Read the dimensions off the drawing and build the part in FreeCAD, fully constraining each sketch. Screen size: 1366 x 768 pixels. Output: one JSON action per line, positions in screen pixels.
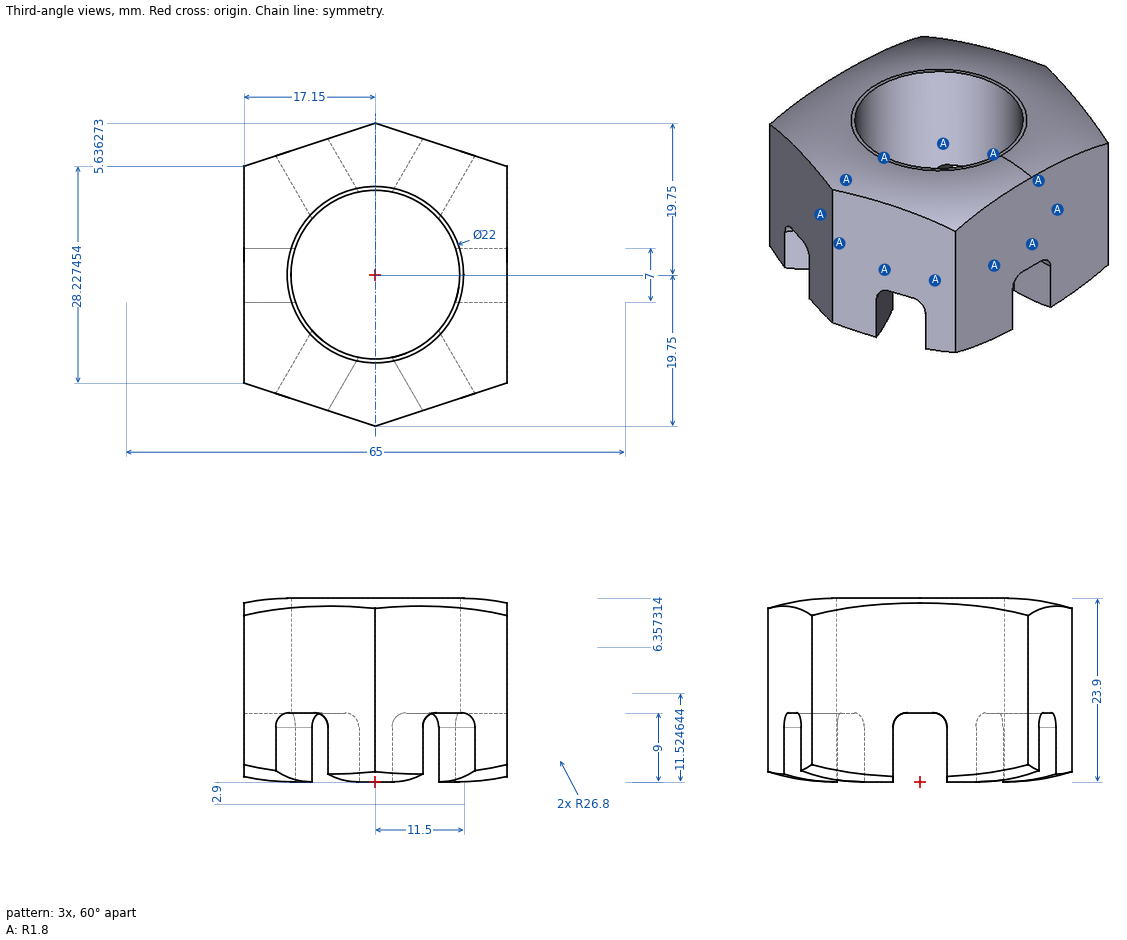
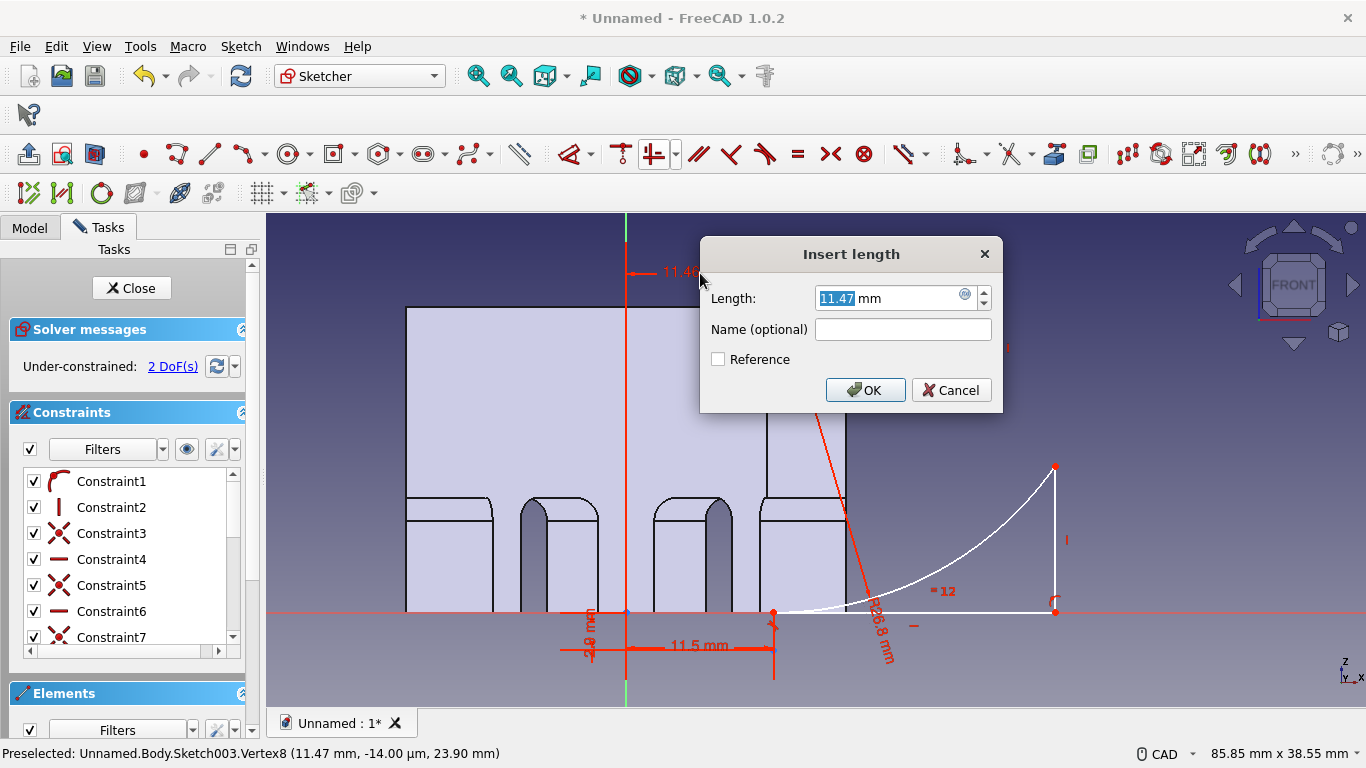
{"action": "type", "text": "11.5"}
{"action": "key", "text": "Return"}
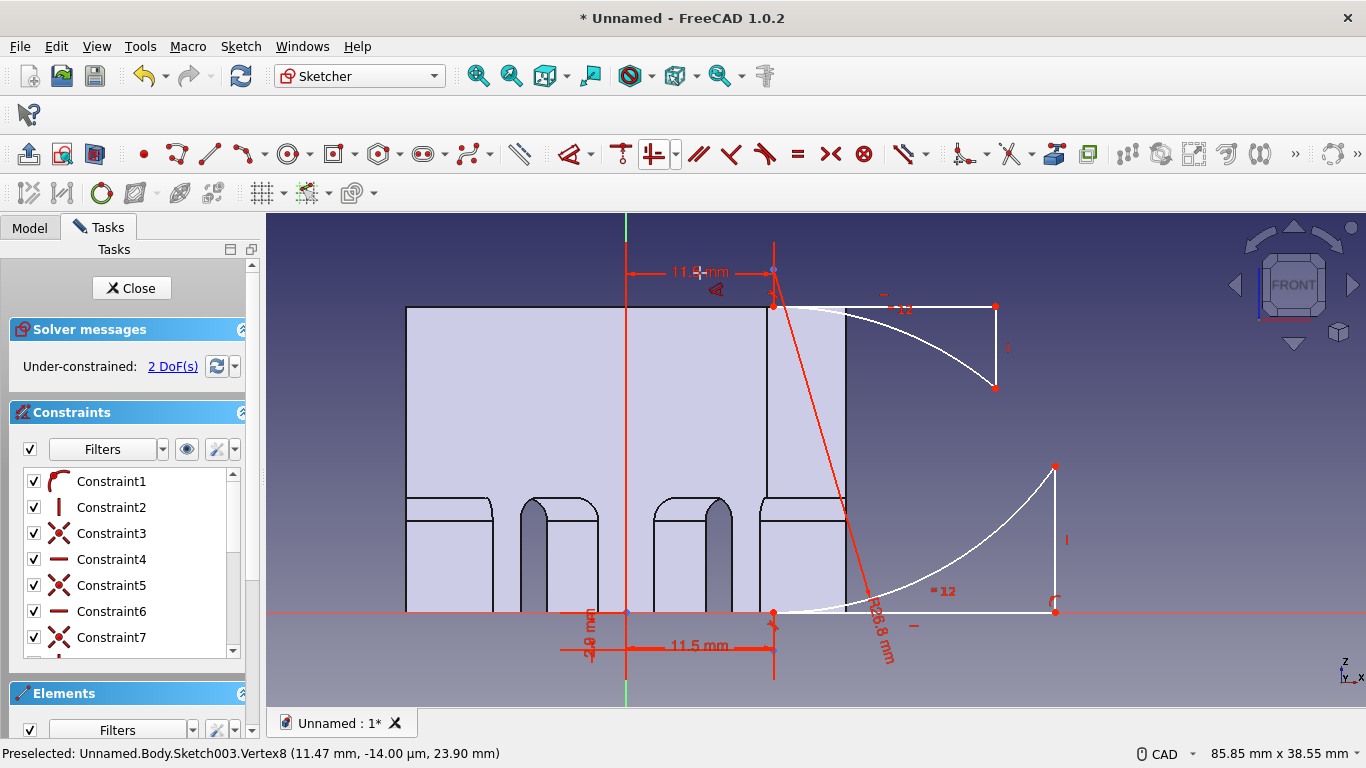
{"action": "left_click", "coordinate": [996, 331]}
{"action": "left_click", "coordinate": [1030, 347]}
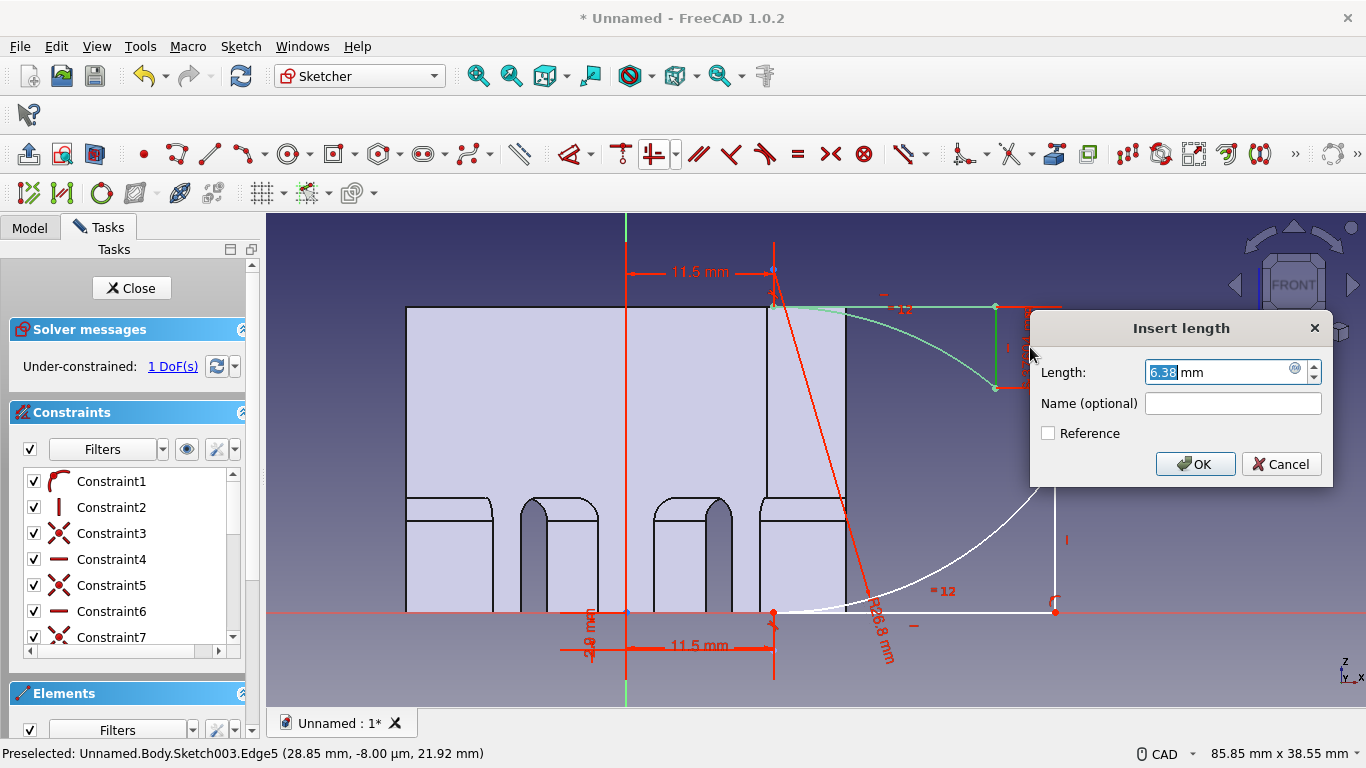
{"action": "type", "text": "6.357314"}
{"action": "key", "text": "Return"}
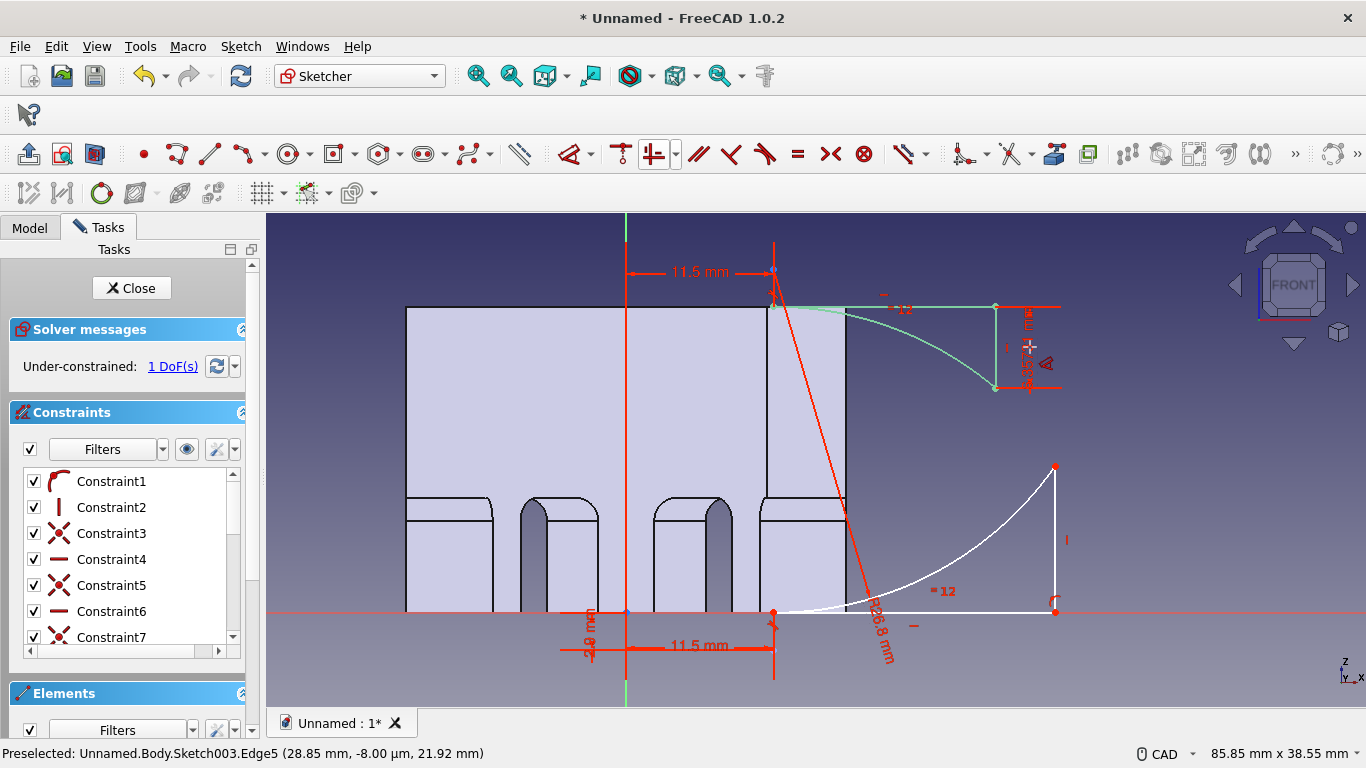
{"action": "left_click", "coordinate": [1055, 510]}
{"action": "left_click", "coordinate": [1089, 540]}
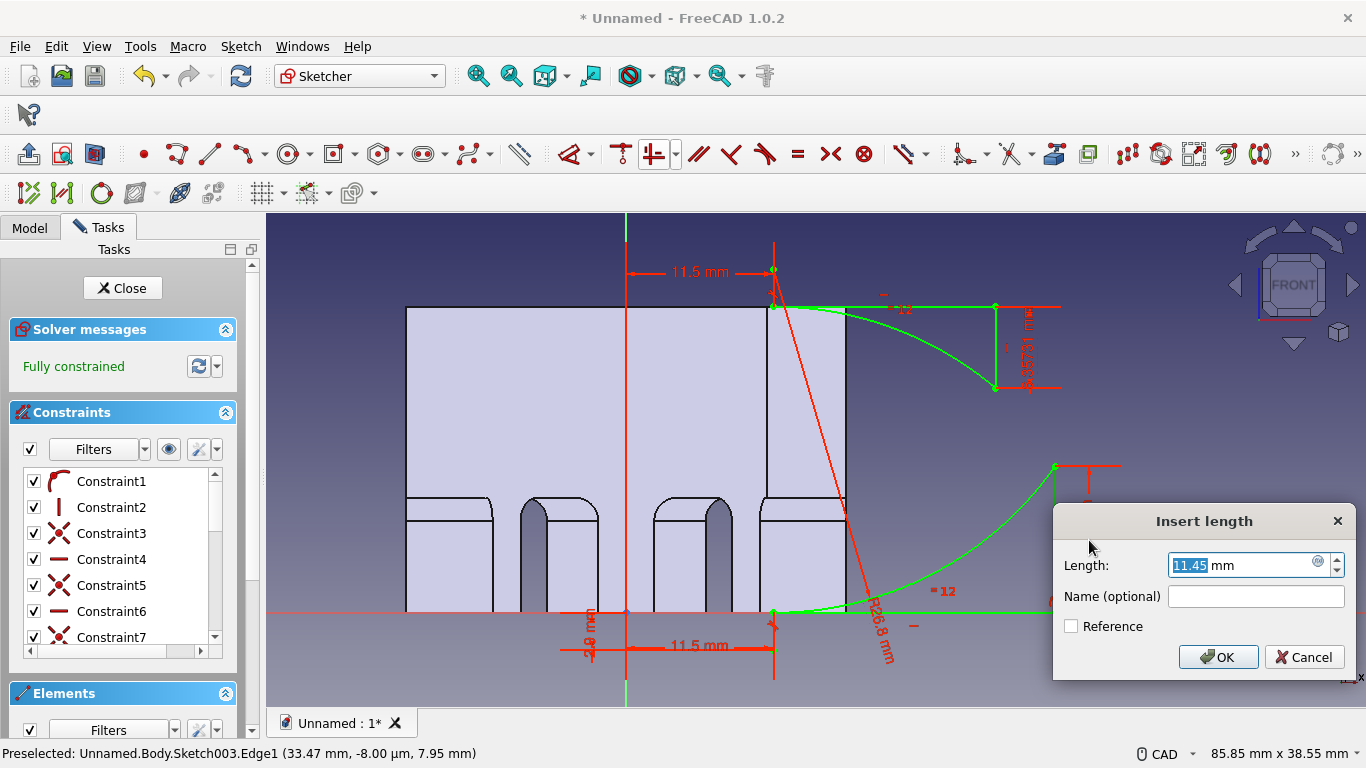
{"action": "type", "text": "11.524644"}
{"action": "key", "text": "Return"}
{"action": "key", "text": "Escape"}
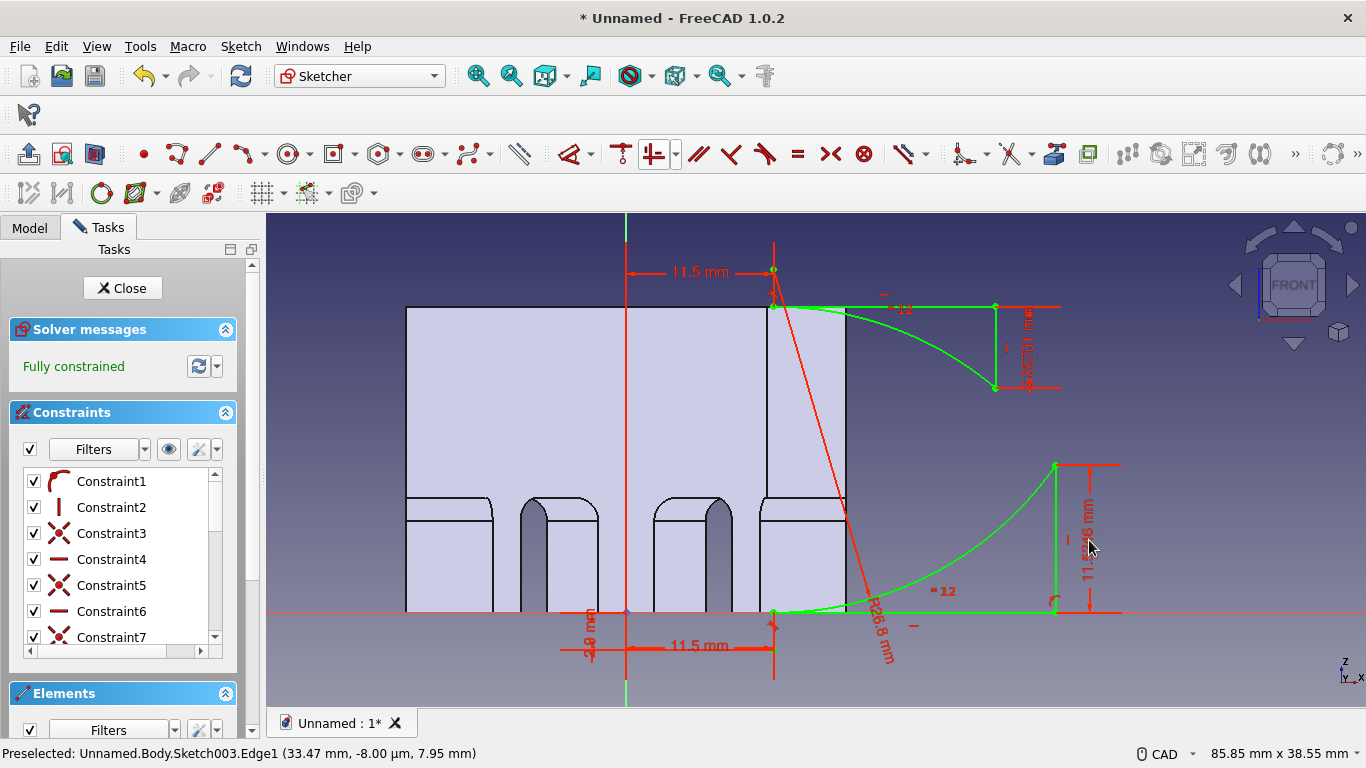
{"action": "left_click", "coordinate": [123, 288]}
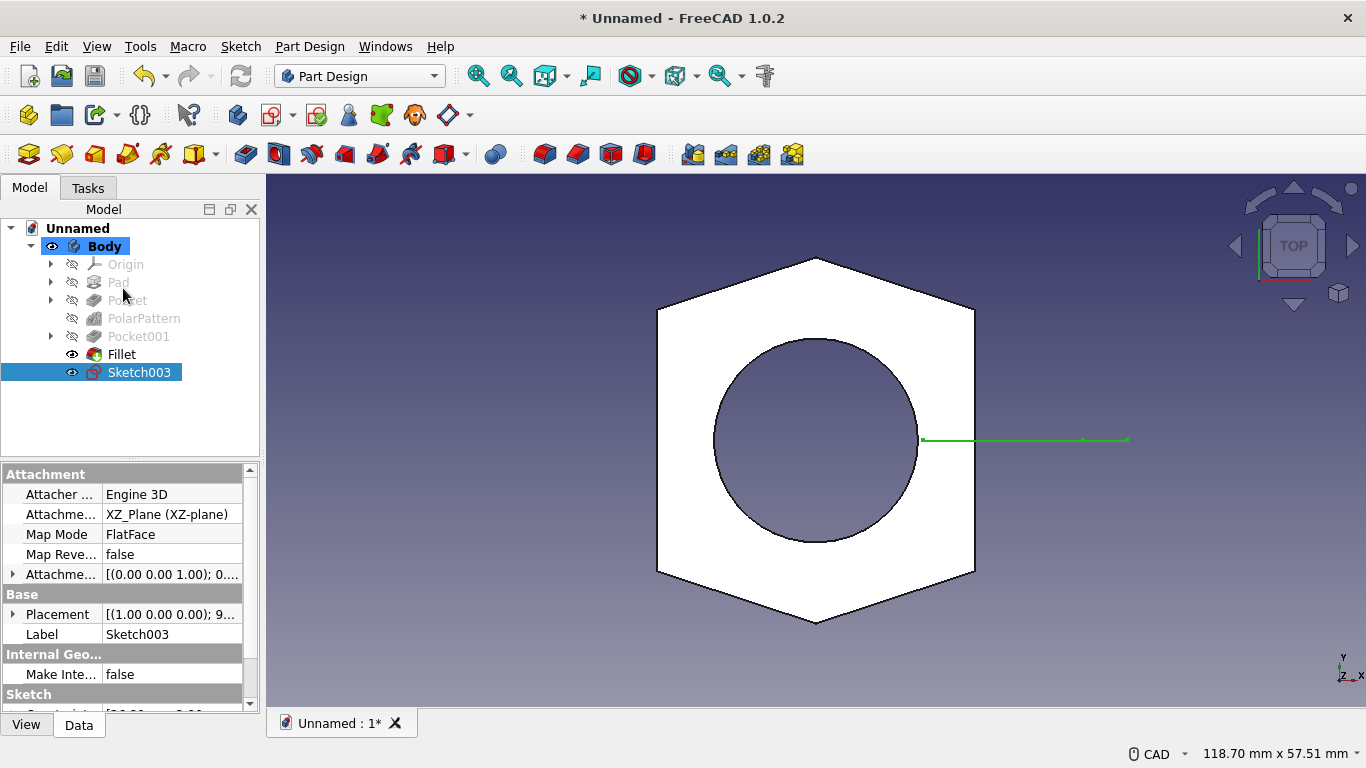
{"action": "left_click", "coordinate": [312, 154]}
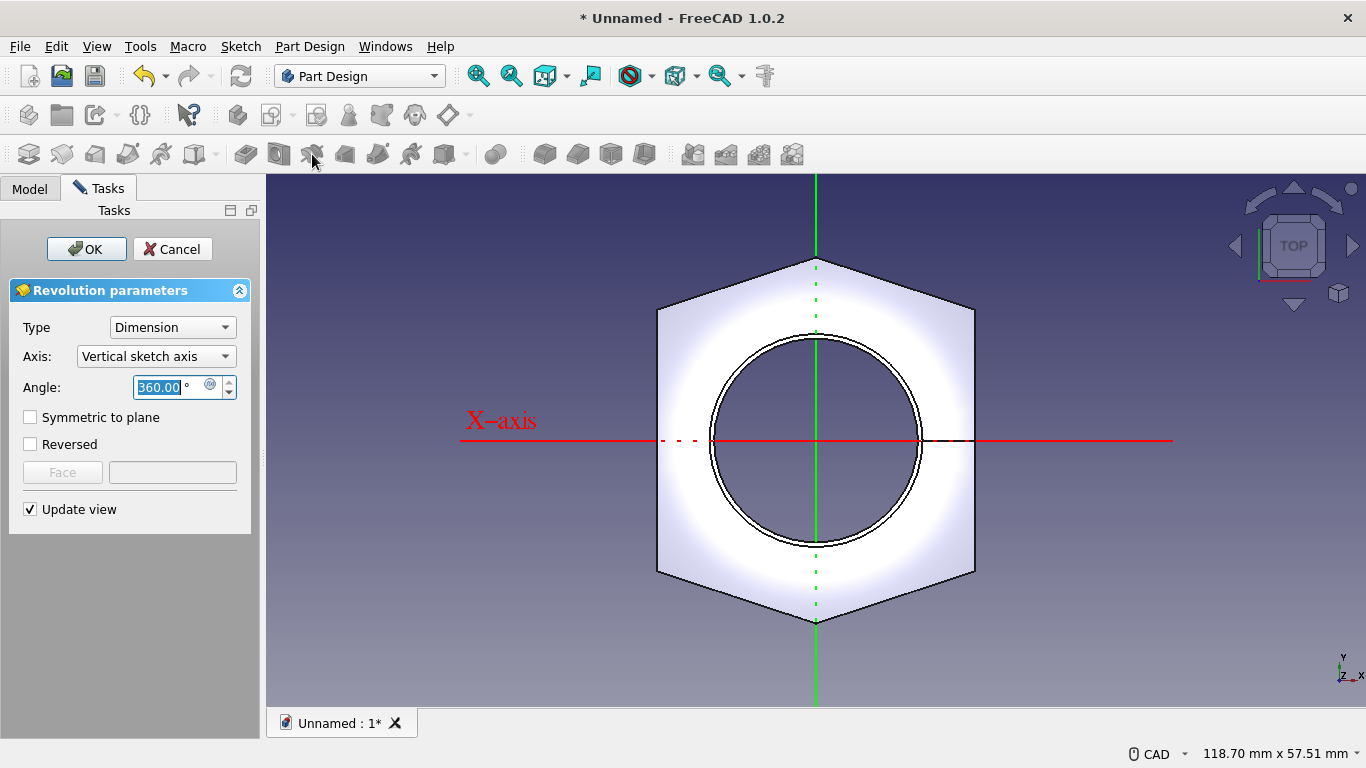
{"action": "left_click", "coordinate": [87, 249]}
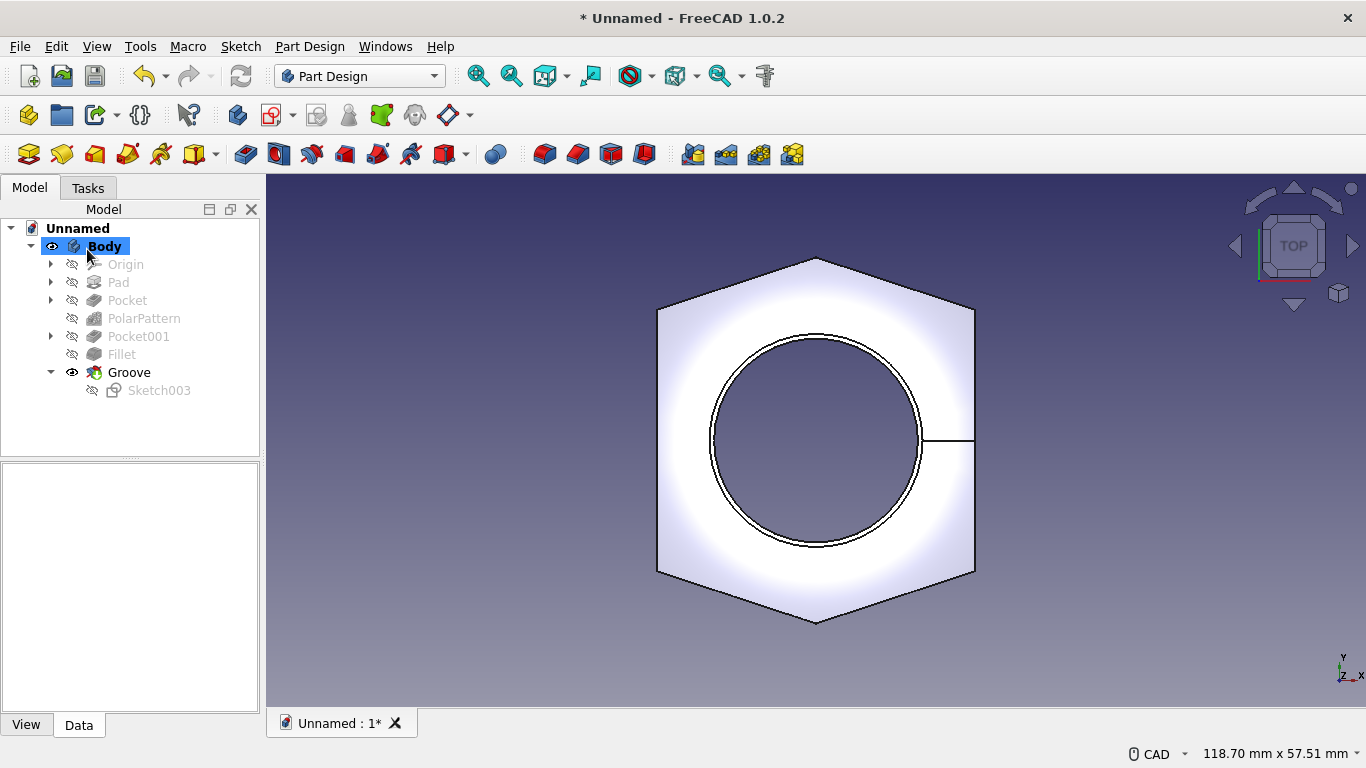
{"action": "key", "text": "0"}